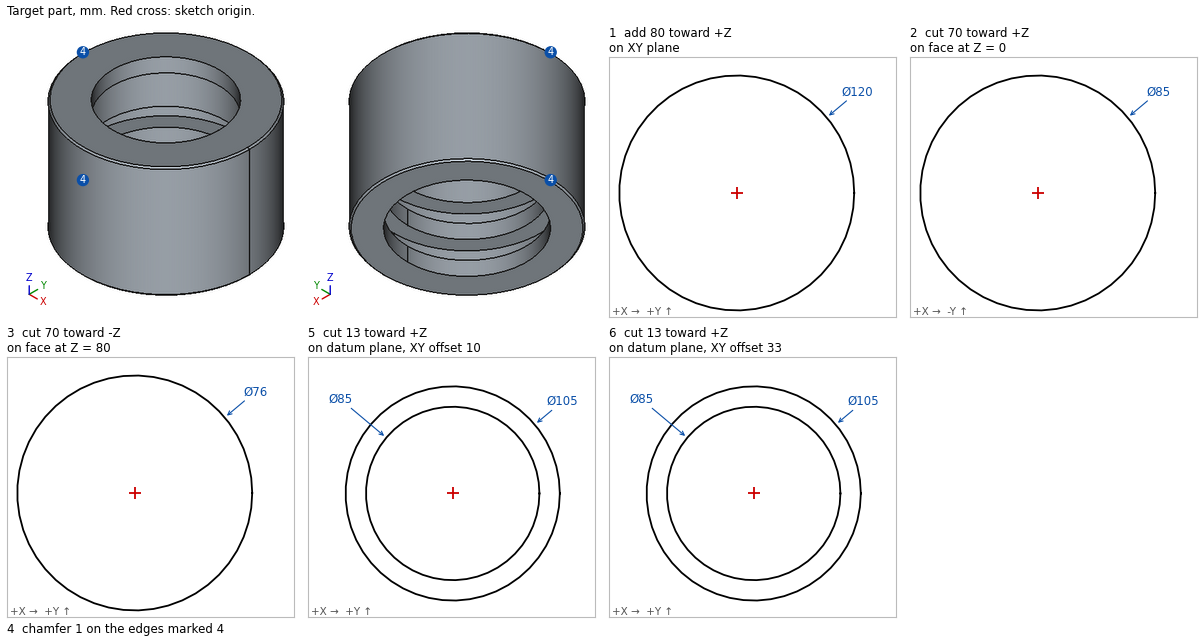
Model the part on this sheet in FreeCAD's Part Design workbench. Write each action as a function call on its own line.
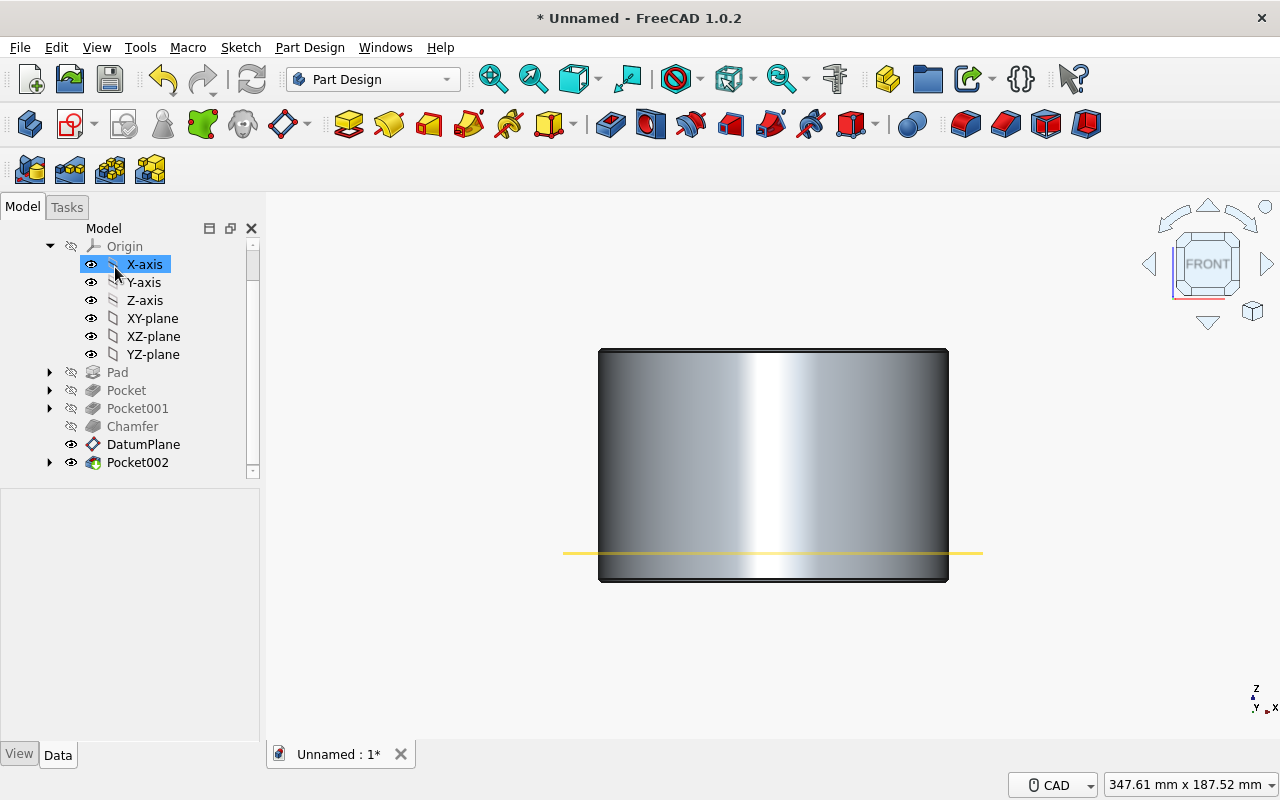
click(116, 444)
key(space)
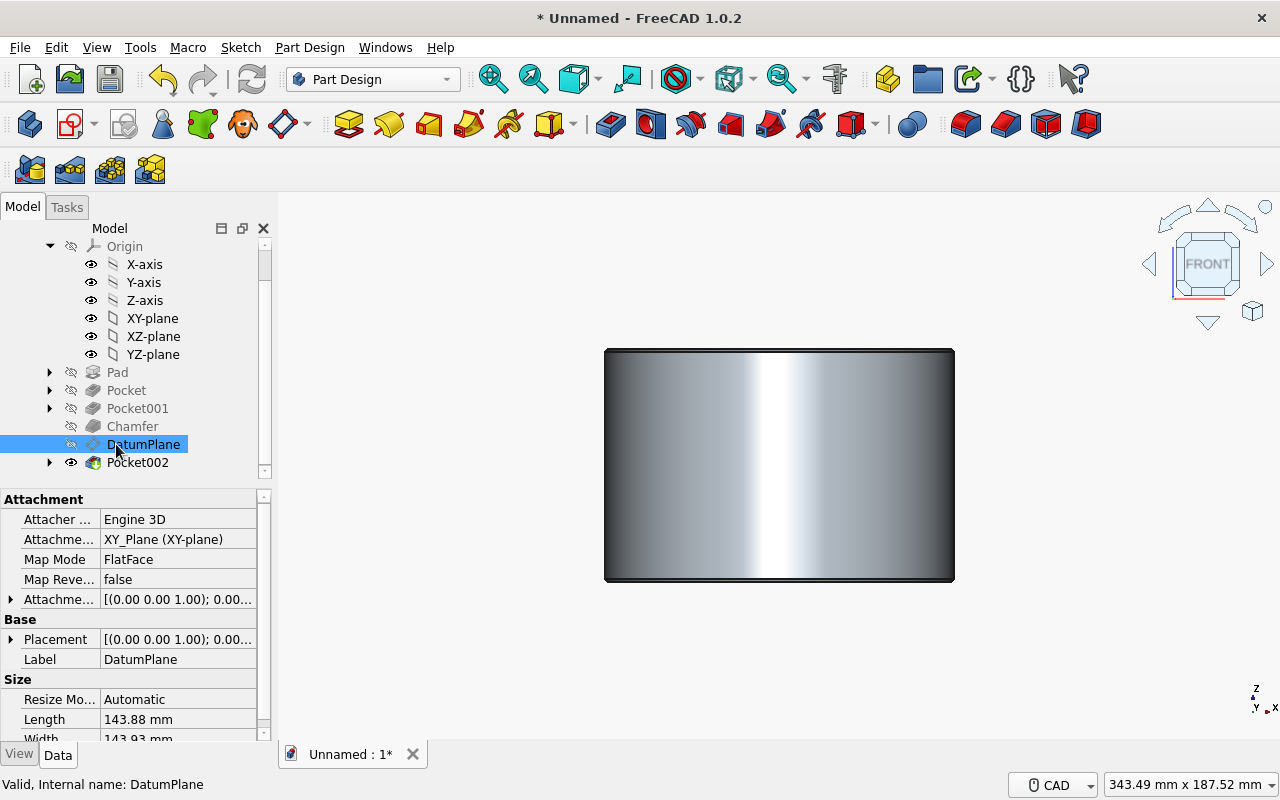
click(494, 80)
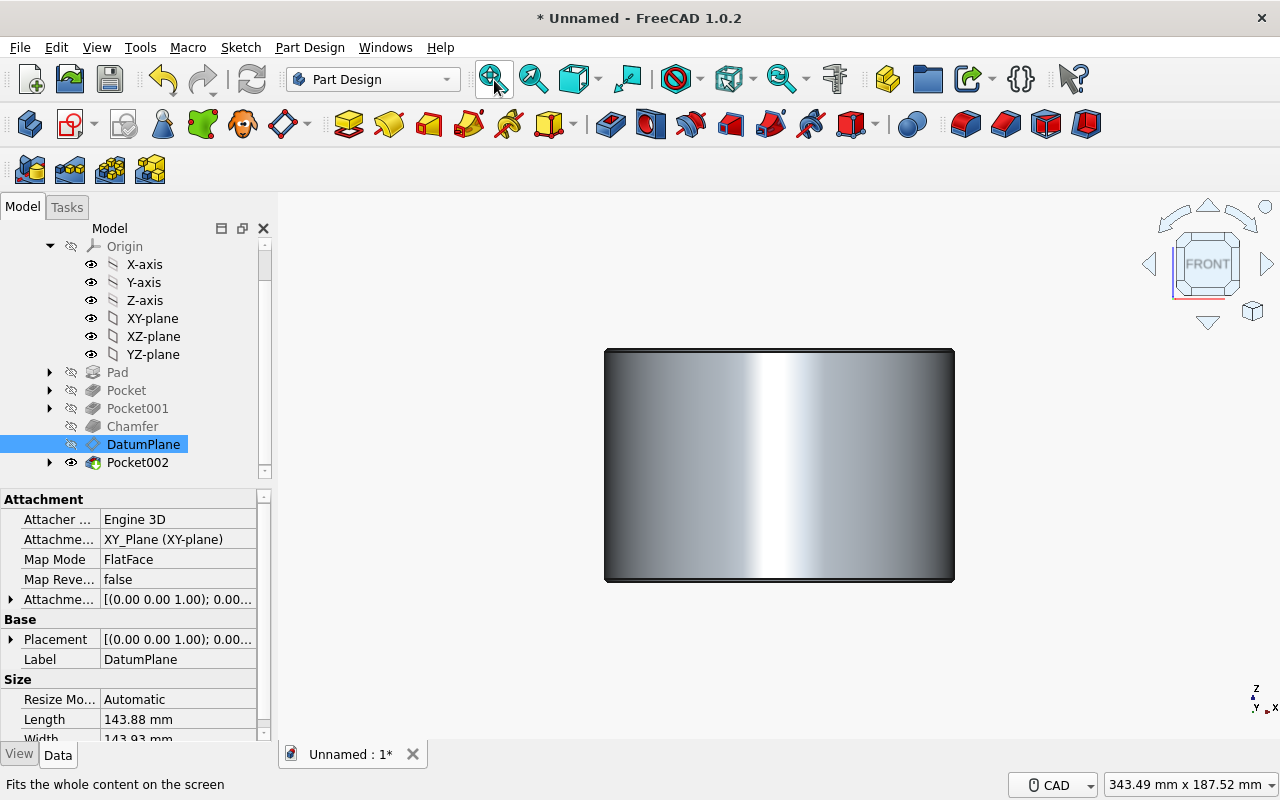
click(136, 318)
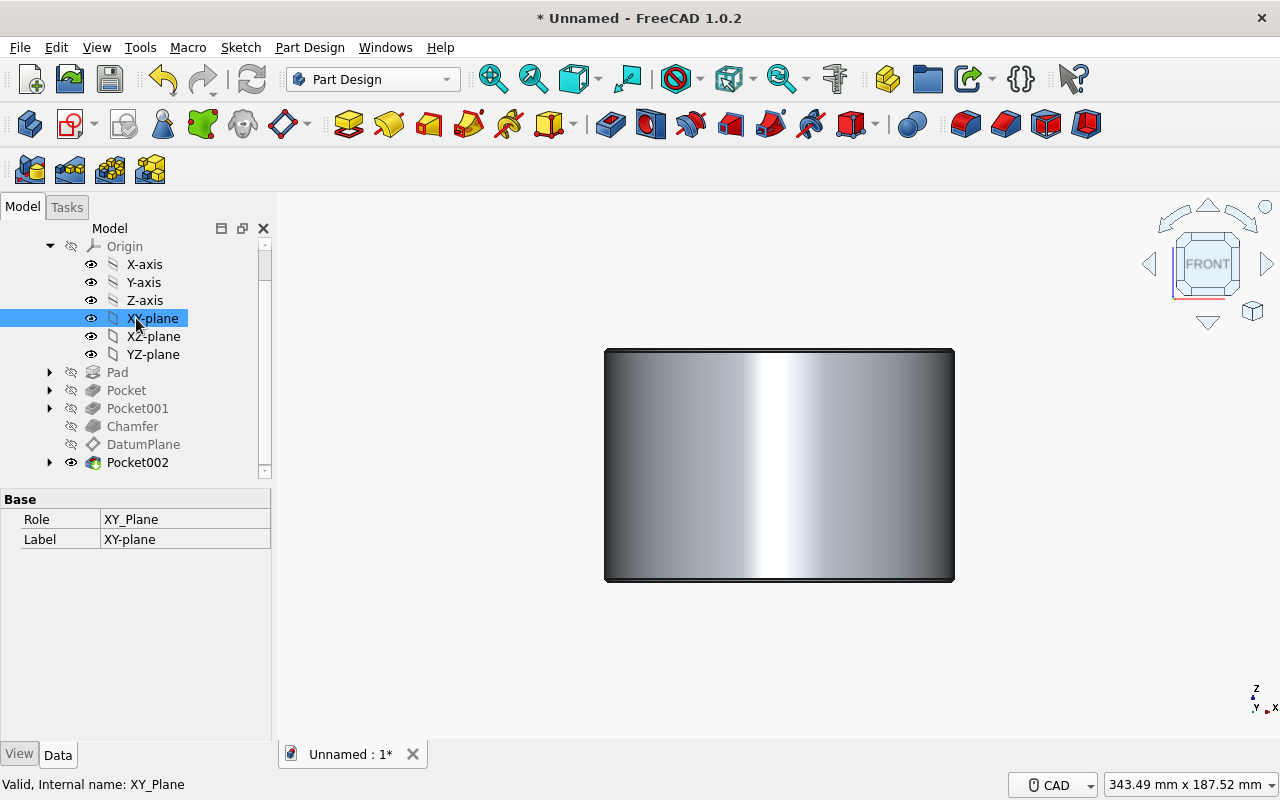
click(284, 124)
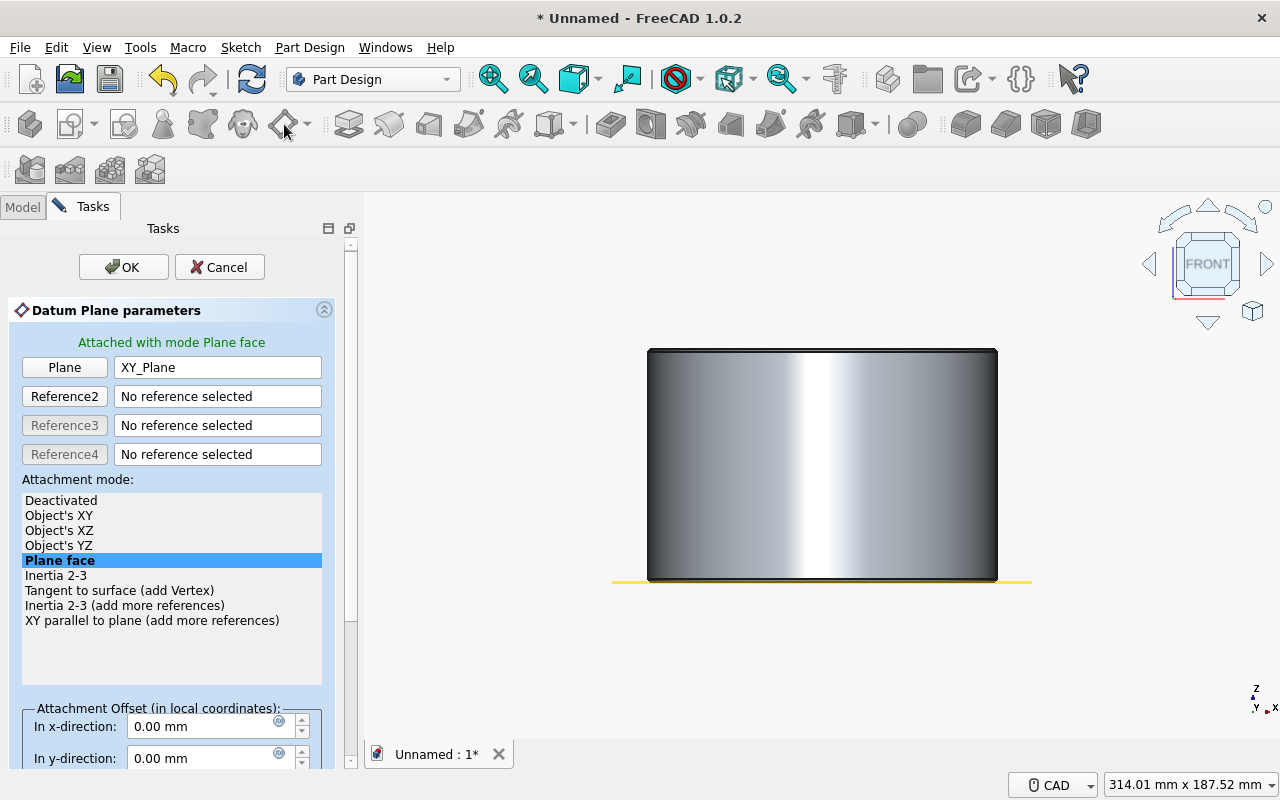
scroll(351, 503, down, 2)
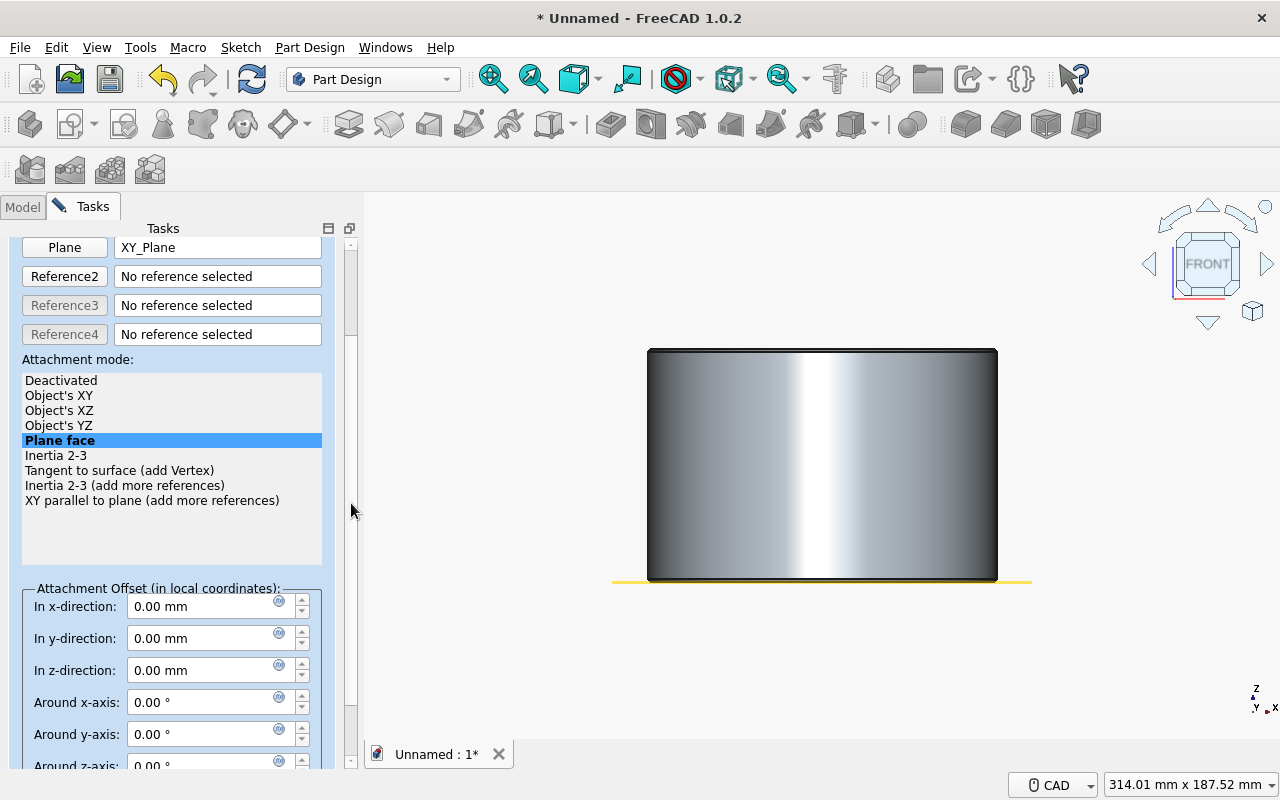
triple_click(210, 670)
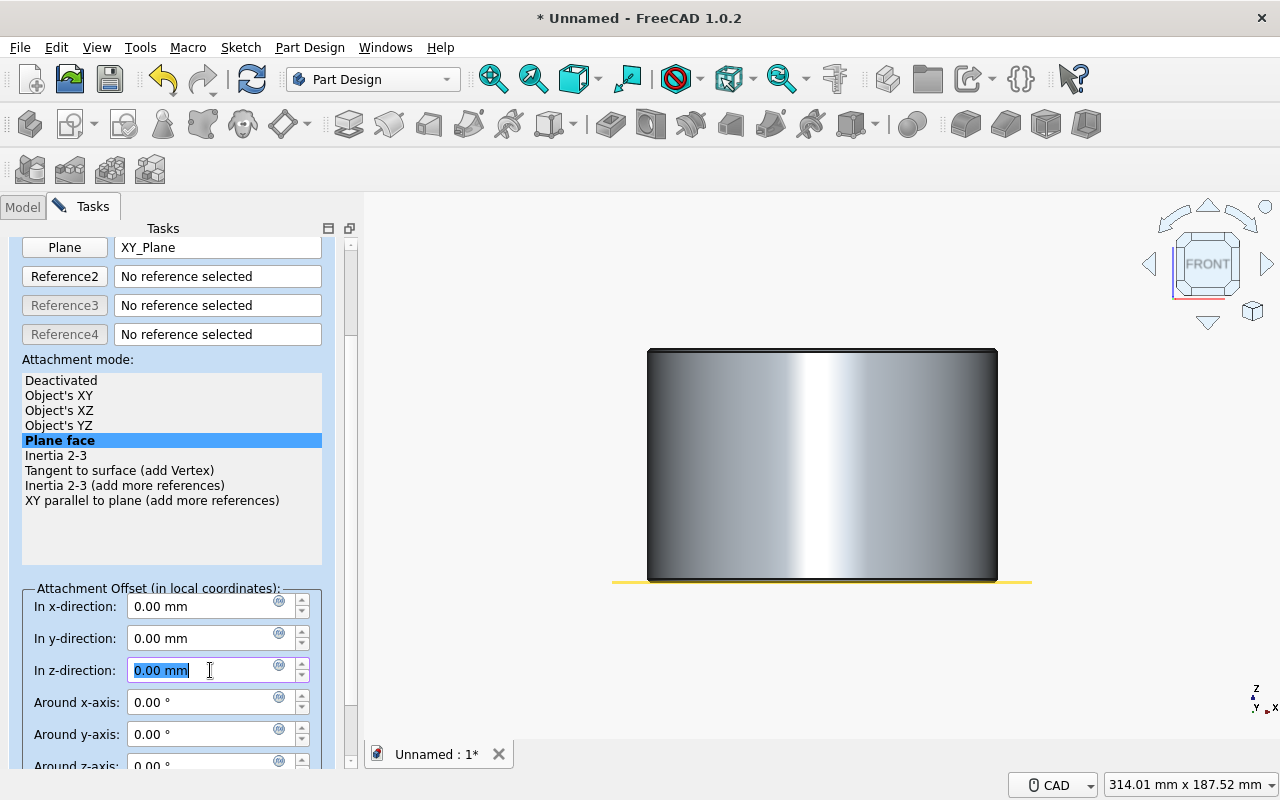
text(33)
key(Tab)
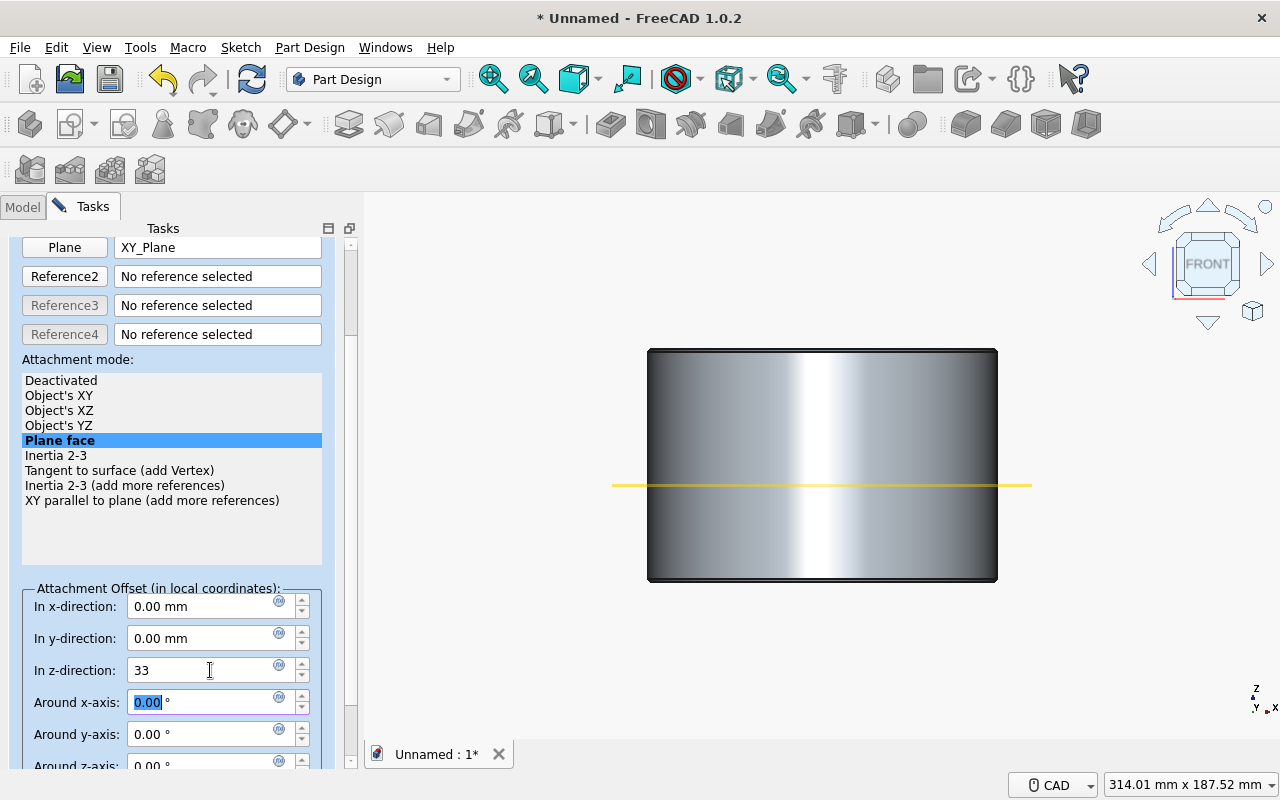
scroll(351, 503, up, 3)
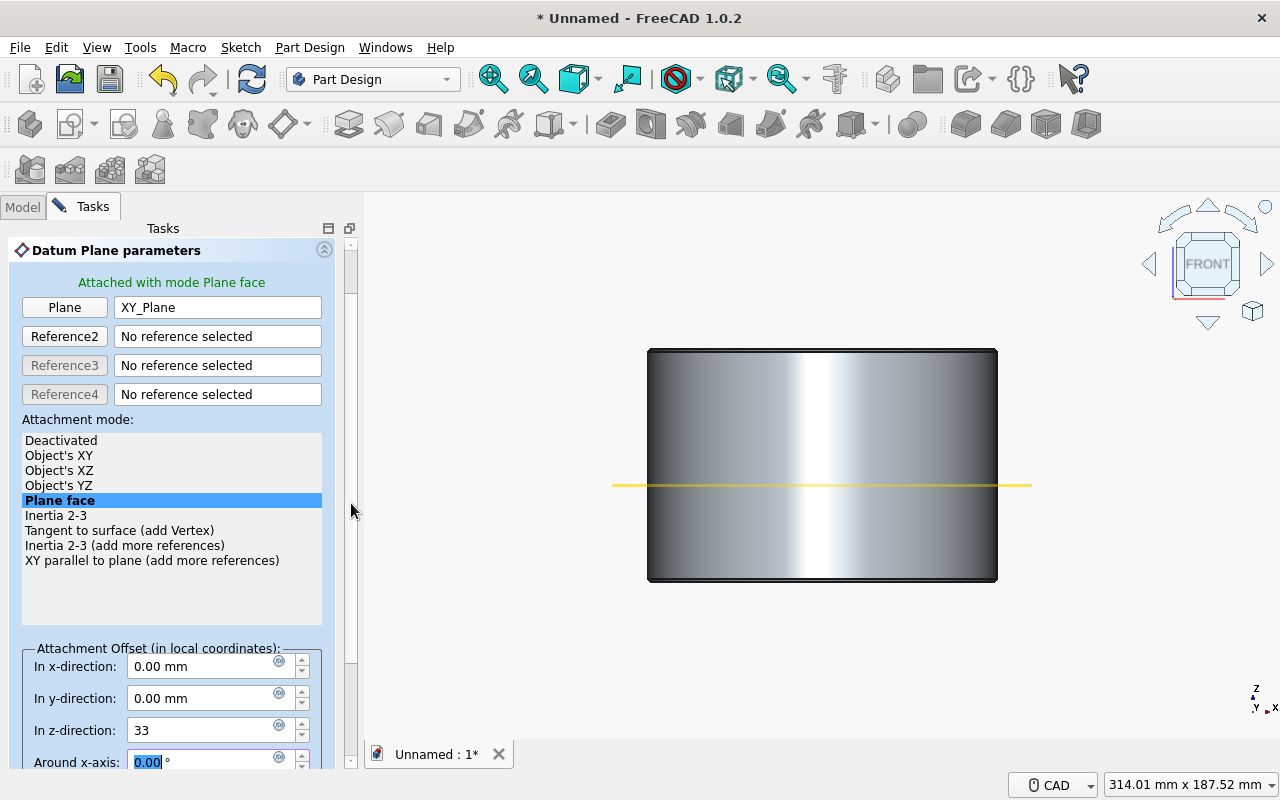
click(124, 267)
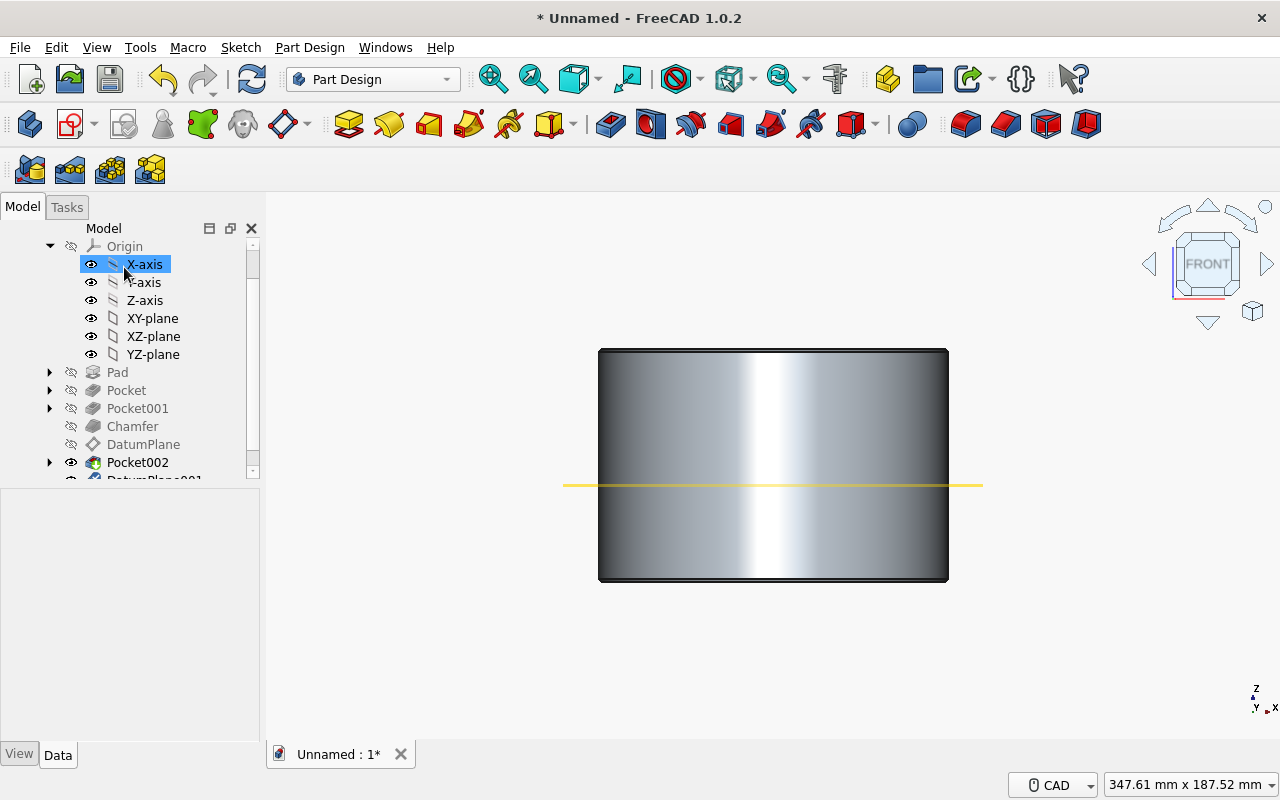
scroll(140, 350, down, 3)